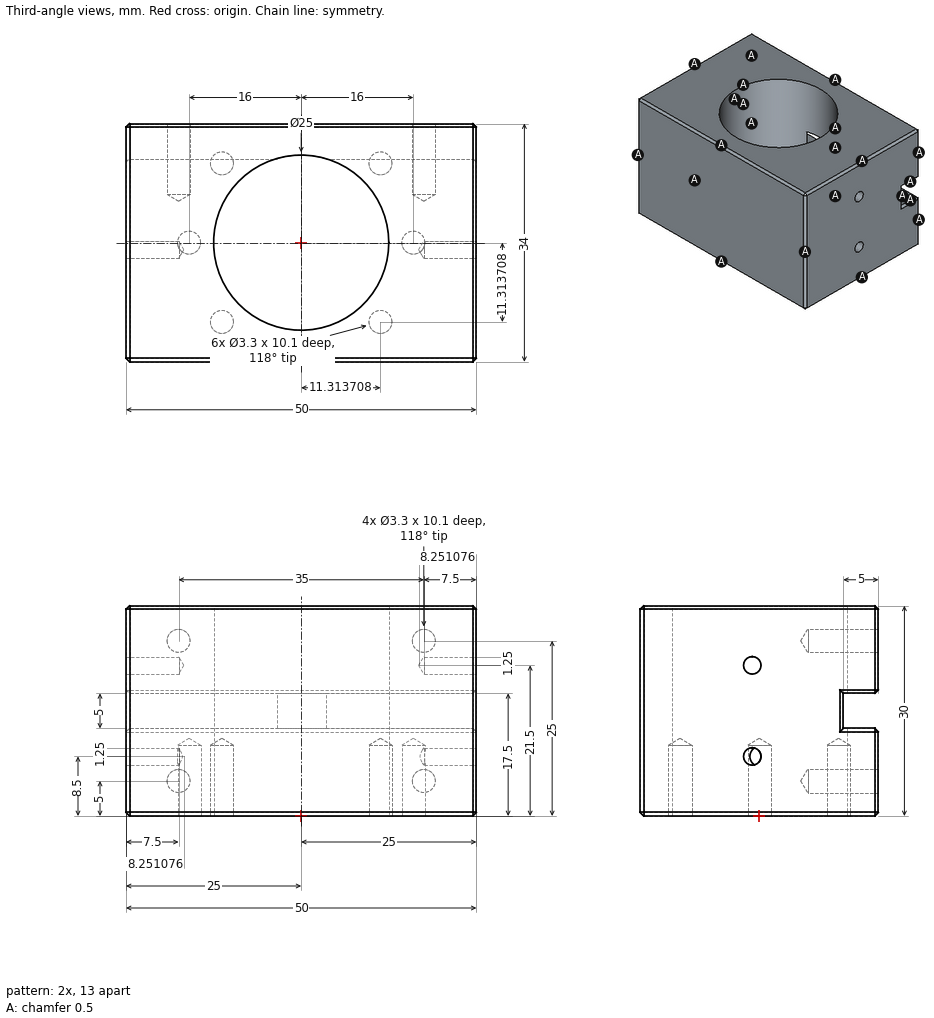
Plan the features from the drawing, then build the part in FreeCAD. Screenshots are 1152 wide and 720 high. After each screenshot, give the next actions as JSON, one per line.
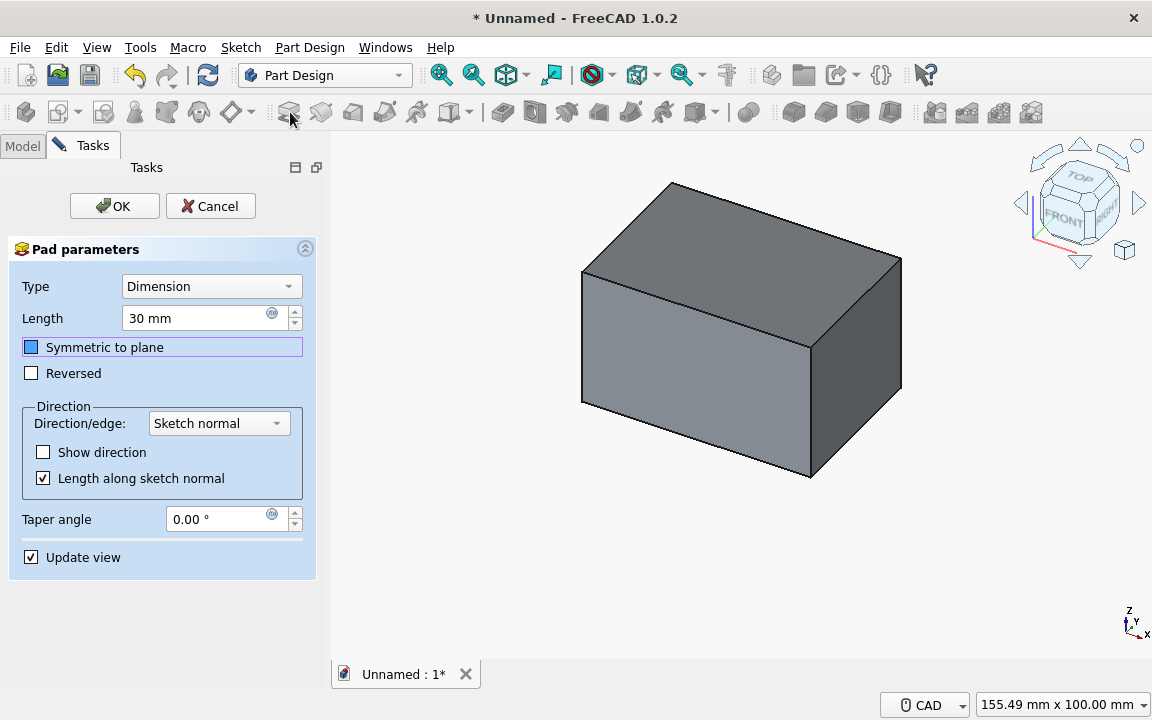
{"action": "left_click", "coordinate": [115, 206]}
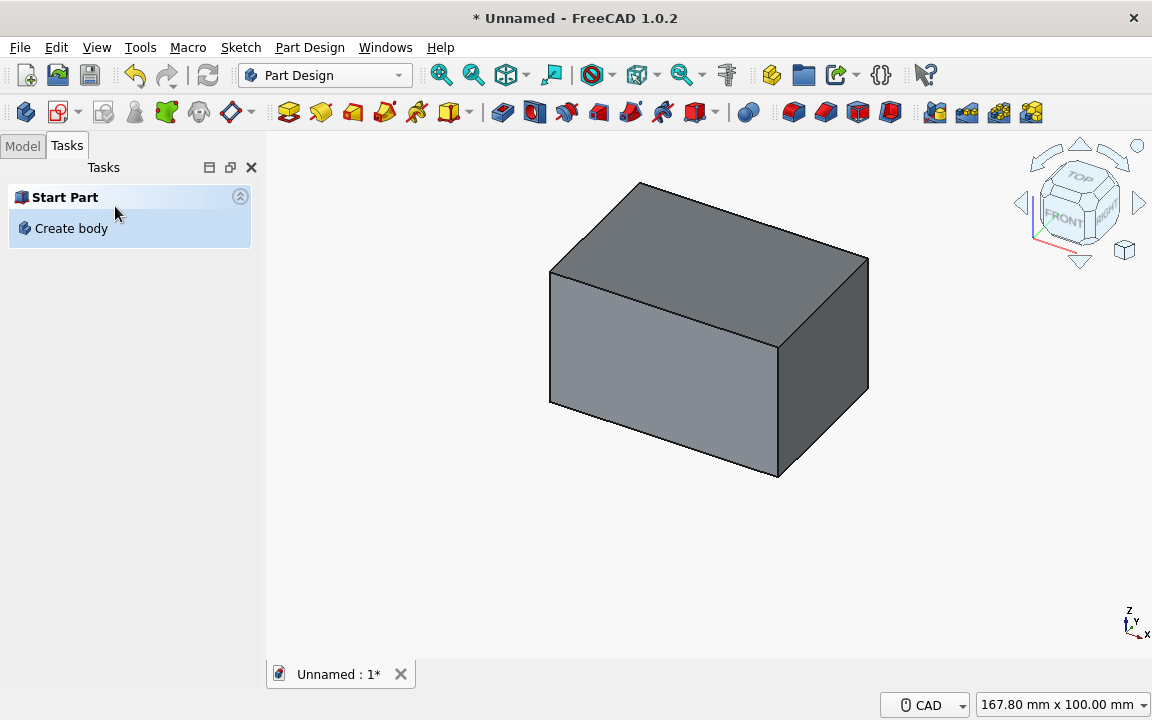
{"action": "left_click", "coordinate": [58, 112]}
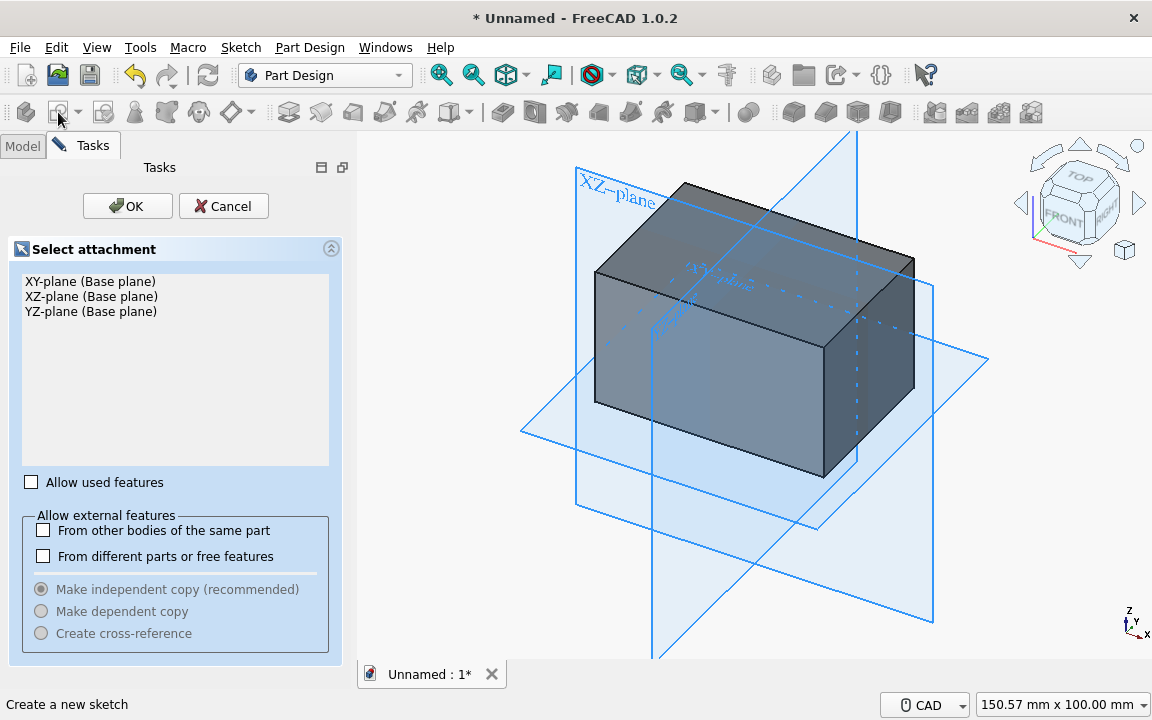
{"action": "left_click", "coordinate": [82, 282]}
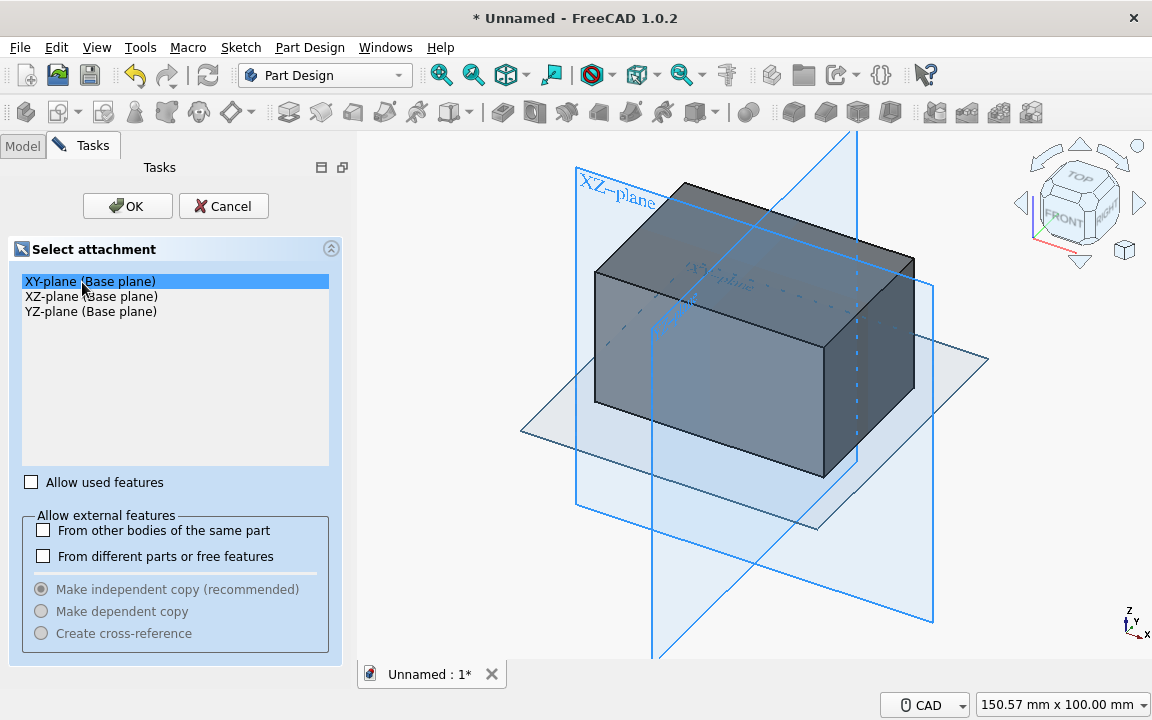
{"action": "left_click", "coordinate": [128, 206]}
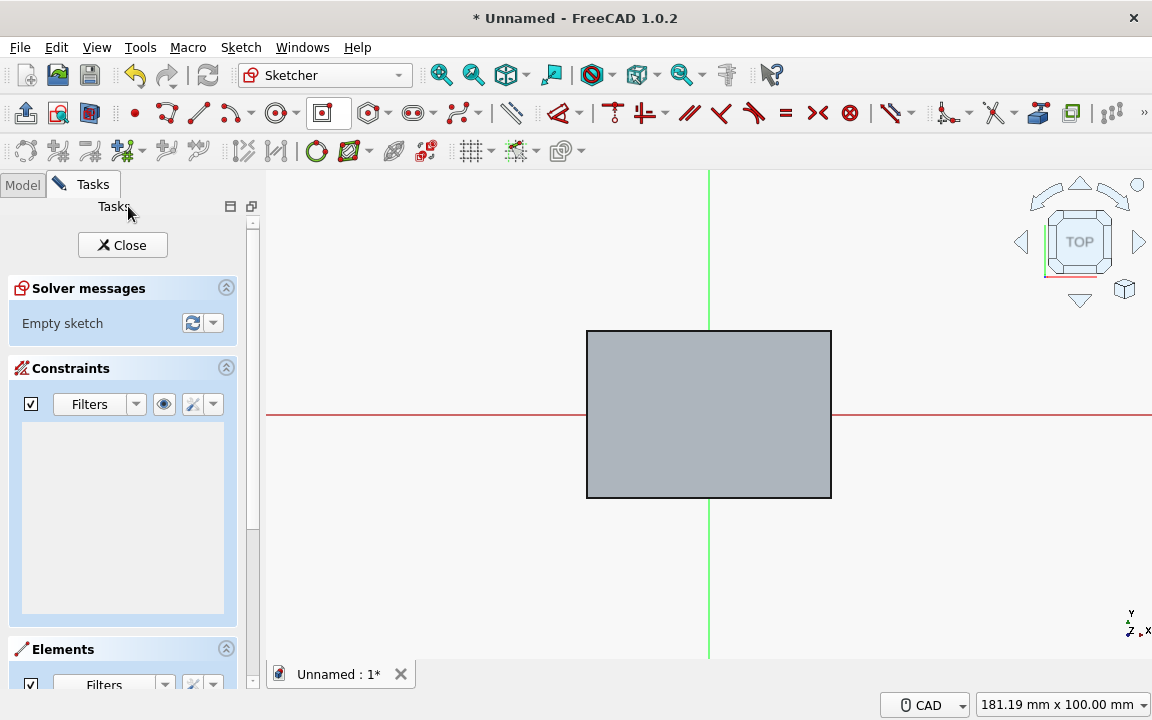
{"action": "key", "text": "q s"}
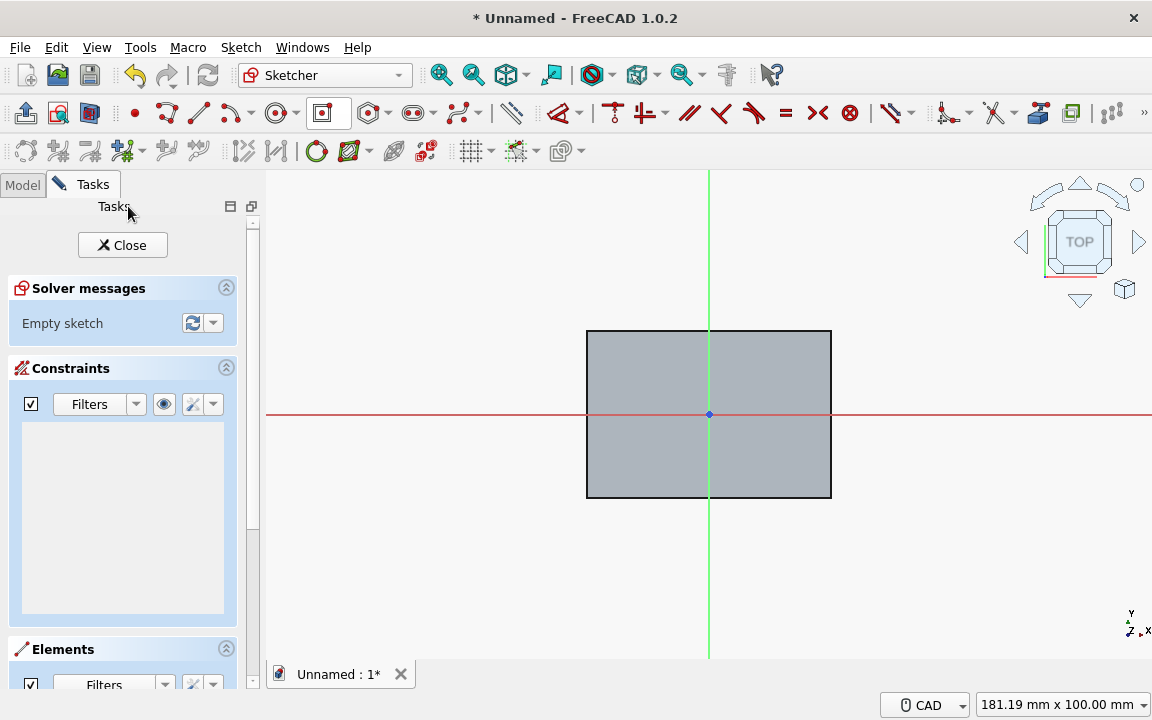
{"action": "scroll", "coordinate": [765, 414], "scroll_direction": "up", "scroll_amount": 4}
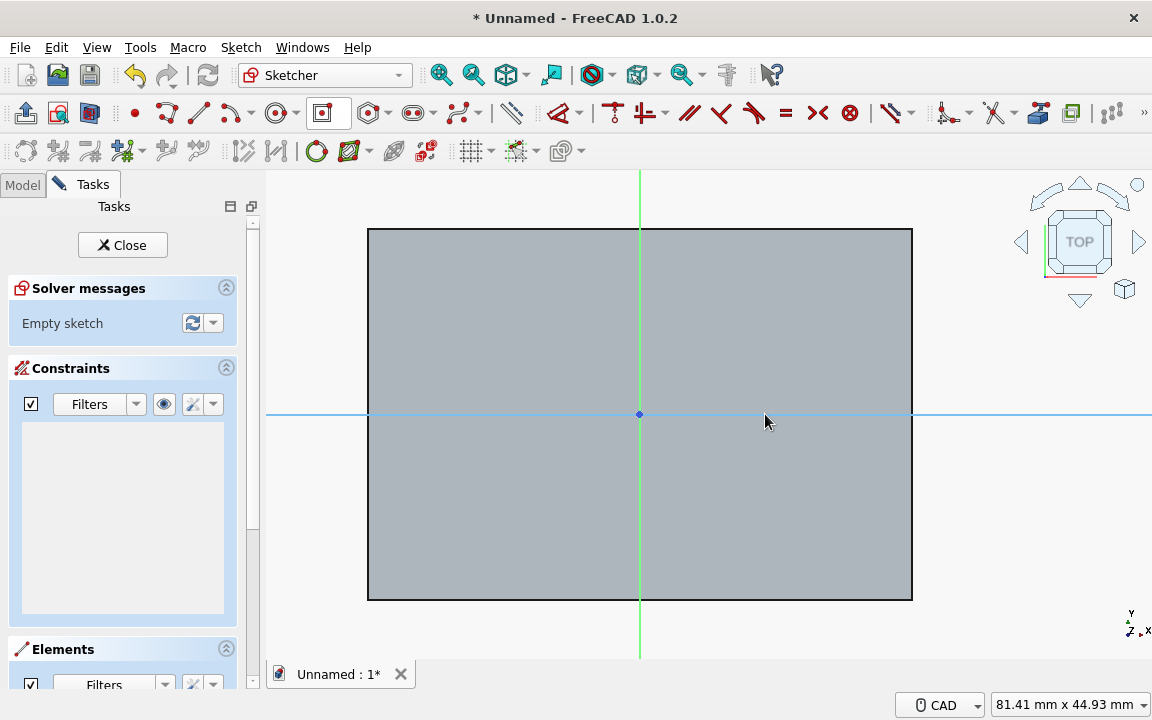
{"action": "key", "text": "g c"}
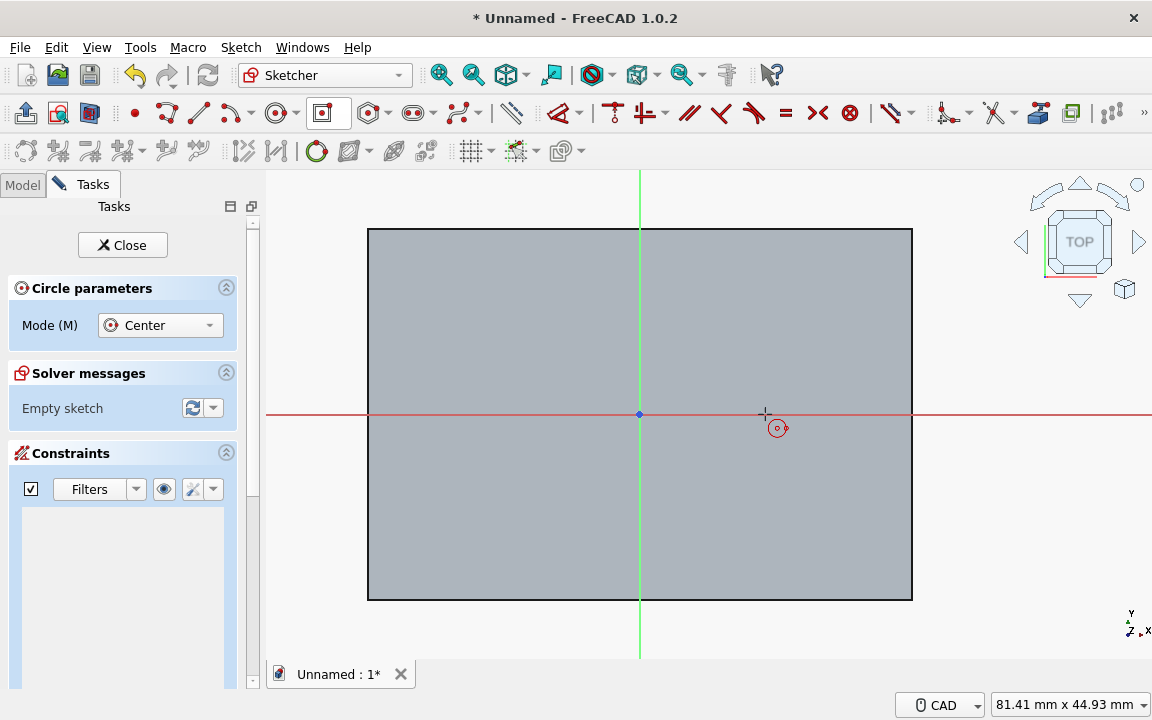
{"action": "scroll", "coordinate": [763, 538], "scroll_direction": "up", "scroll_amount": 2}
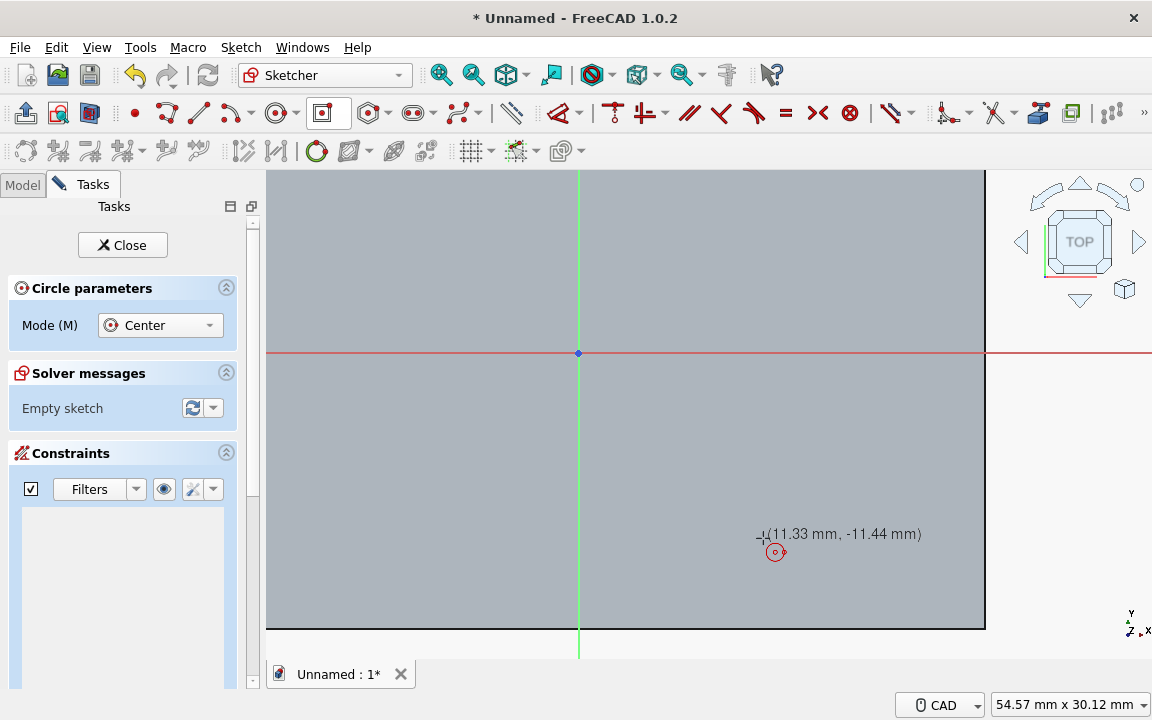
{"action": "left_click", "coordinate": [762, 537]}
{"action": "mouse_move", "coordinate": [781, 518]}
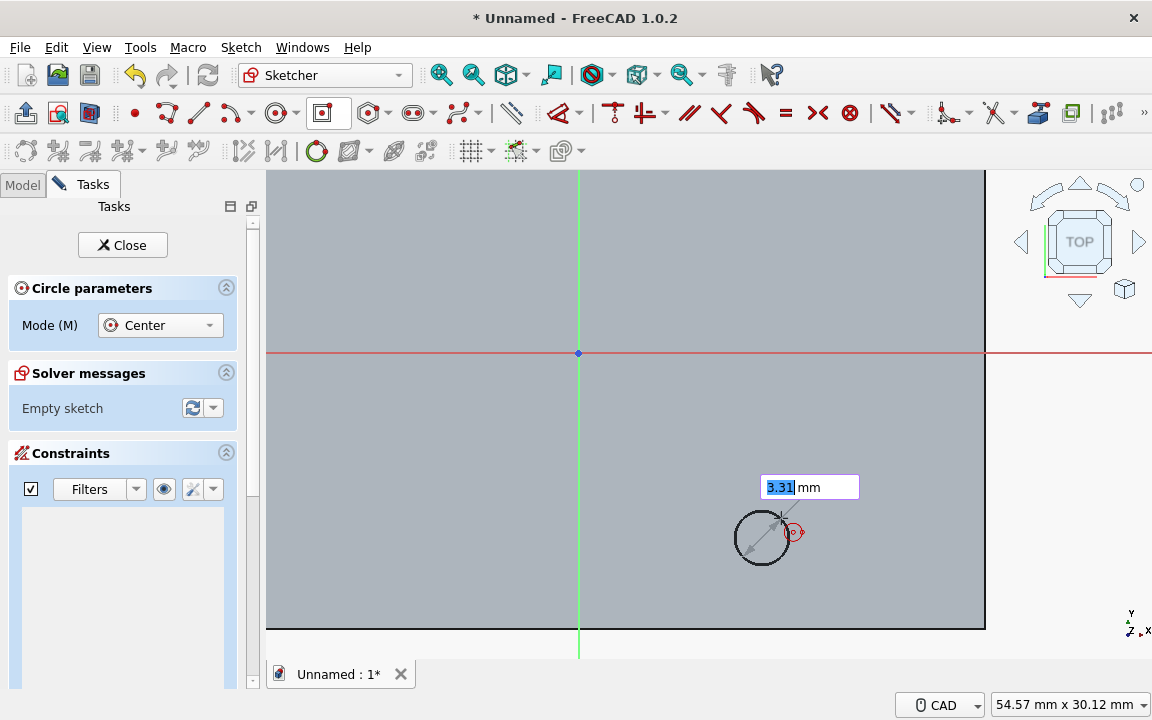
{"action": "type", "text": "3.3"}
{"action": "key", "text": "Return"}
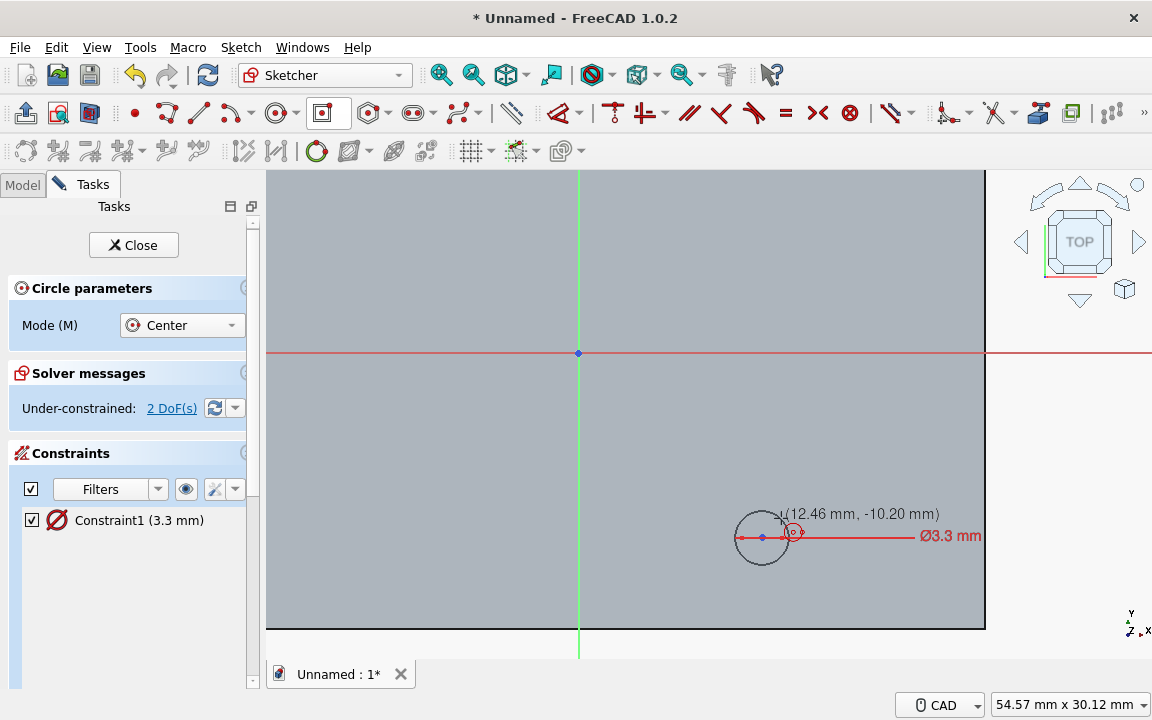
{"action": "left_click", "coordinate": [839, 353]}
{"action": "mouse_move", "coordinate": [857, 334]}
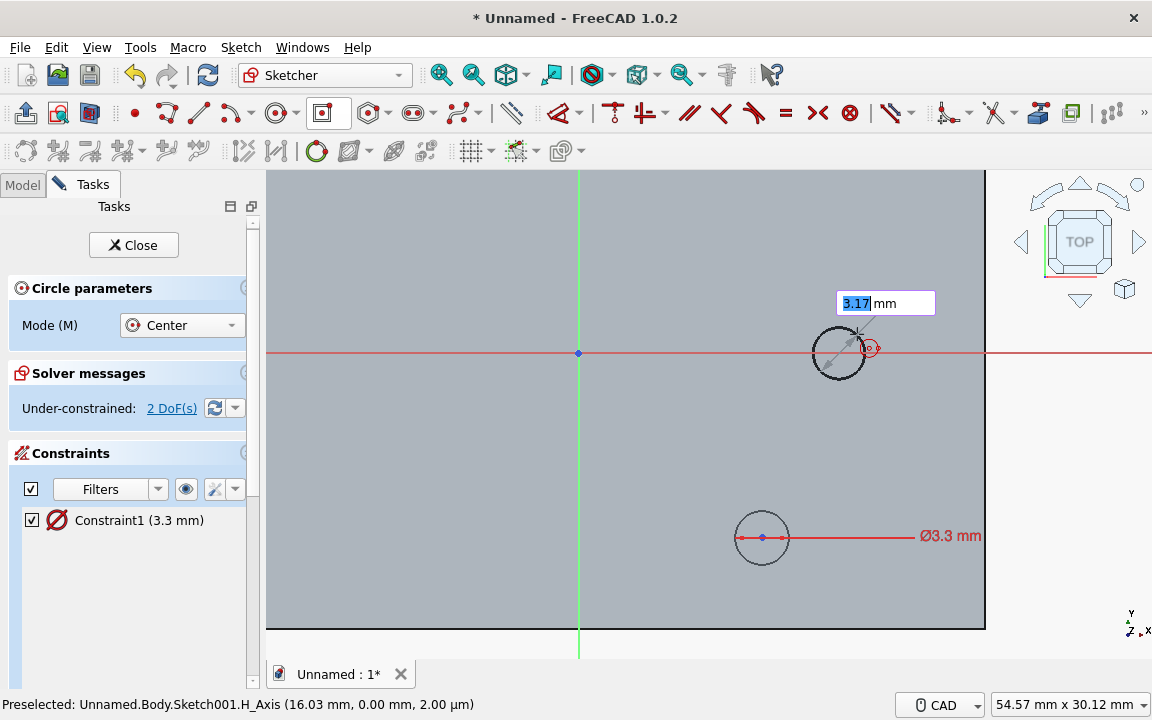
{"action": "type", "text": "3.3"}
{"action": "key", "text": "Return"}